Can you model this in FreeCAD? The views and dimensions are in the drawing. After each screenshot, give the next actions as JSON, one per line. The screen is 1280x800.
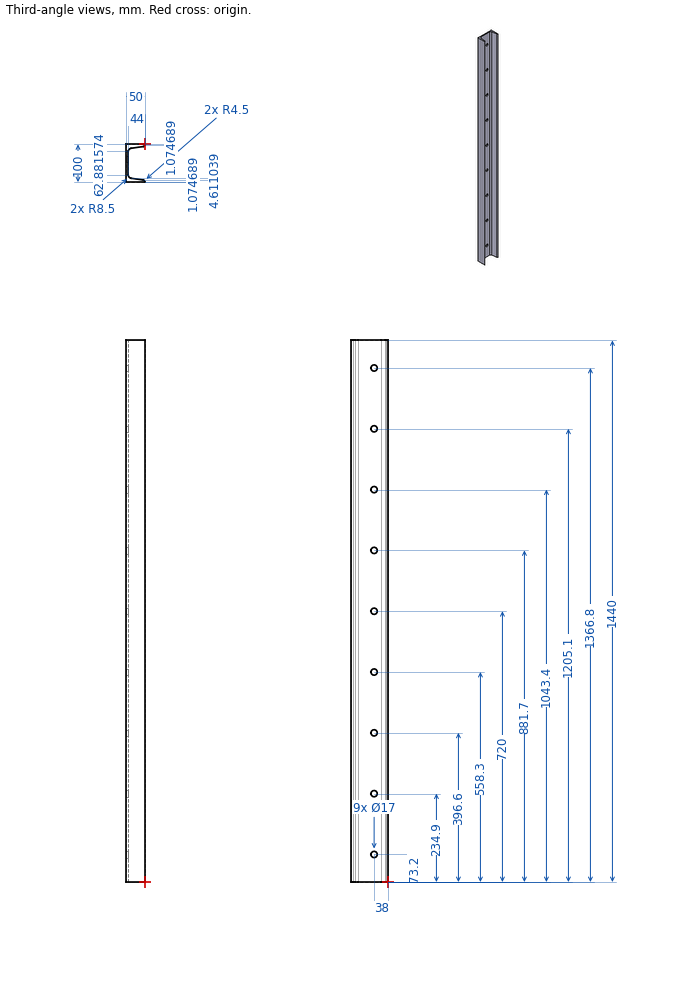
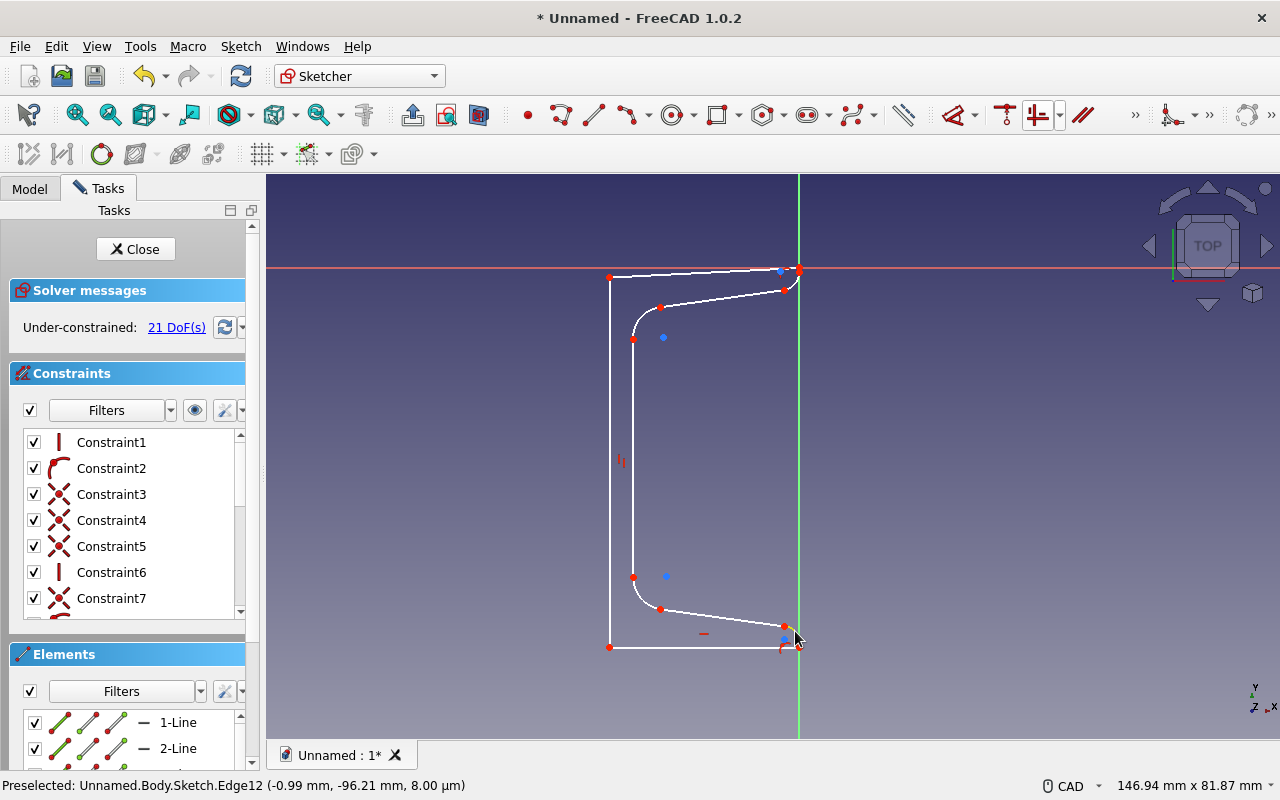
{"action": "left_click", "coordinate": [747, 621]}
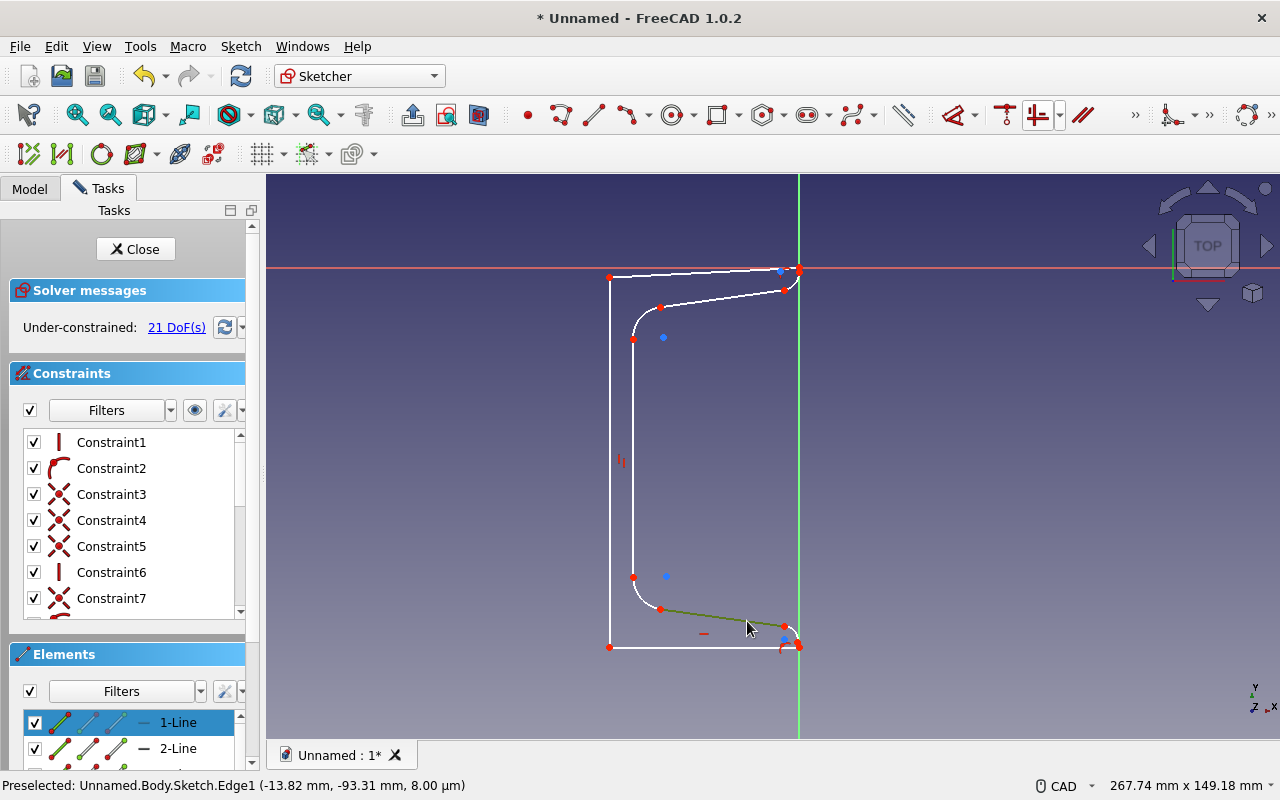
{"action": "left_click", "coordinate": [636, 591]}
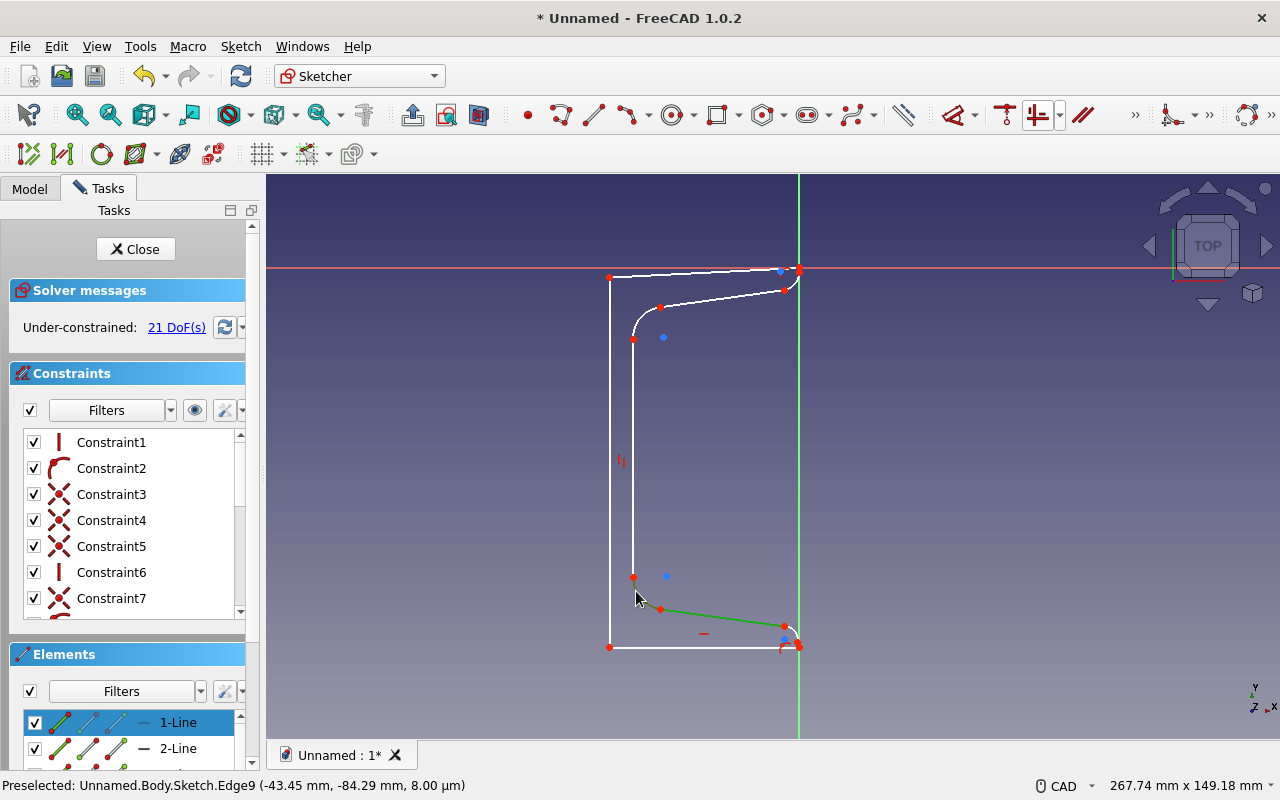
{"action": "key", "text": "t"}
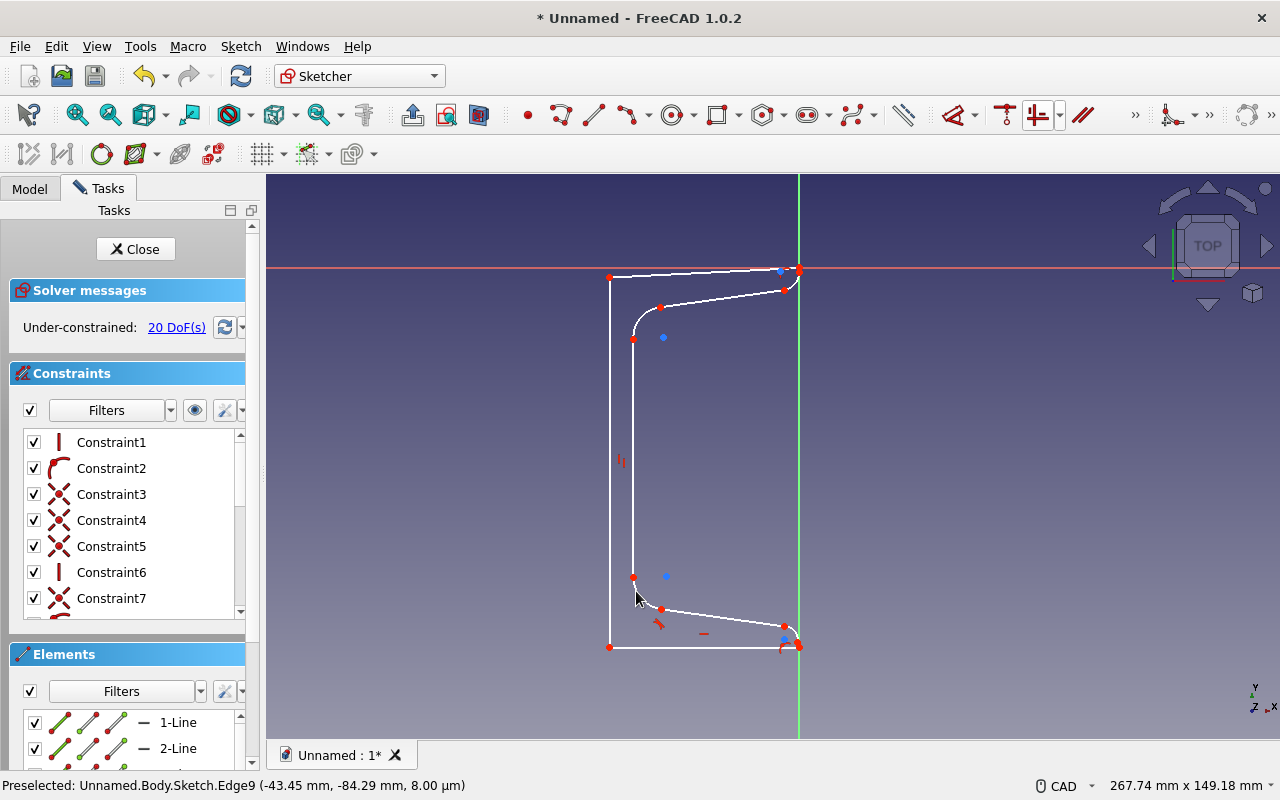
{"action": "left_click", "coordinate": [748, 621]}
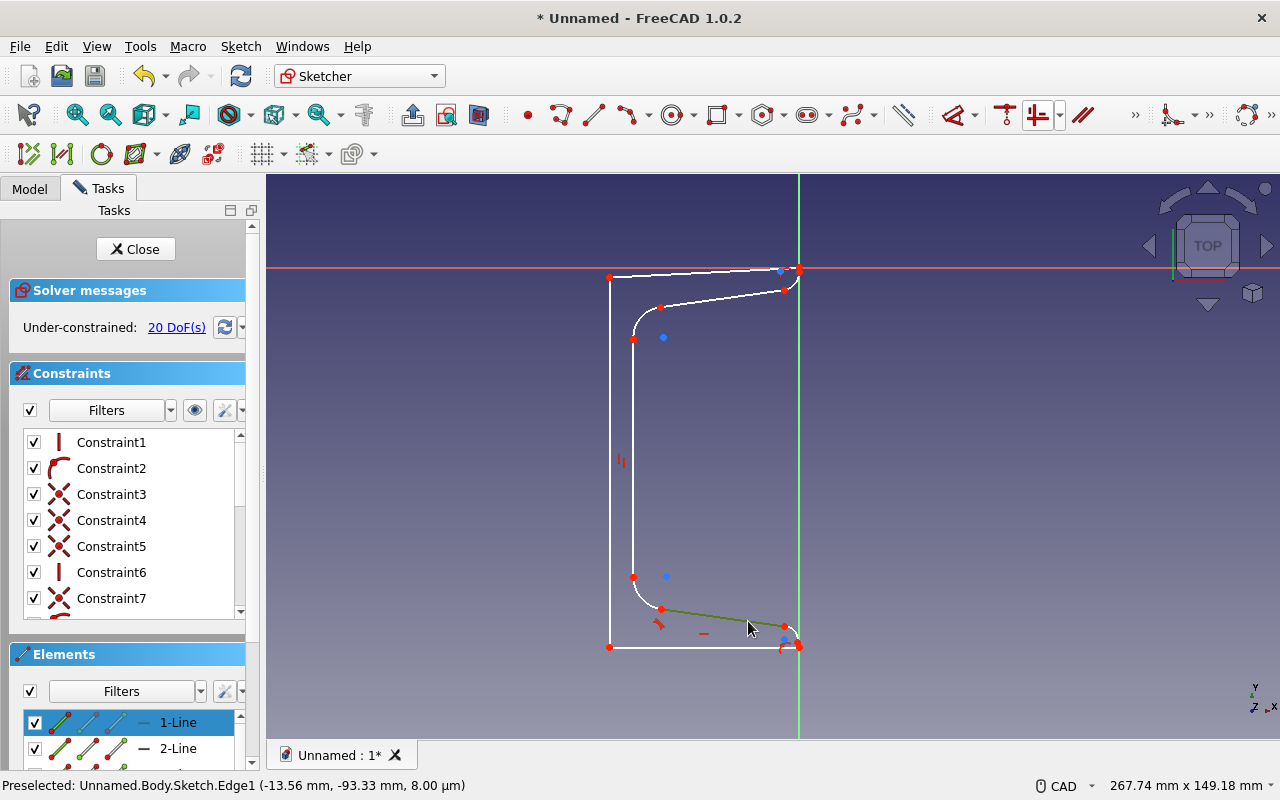
{"action": "scroll", "coordinate": [792, 628], "scroll_direction": "up", "scroll_amount": 4}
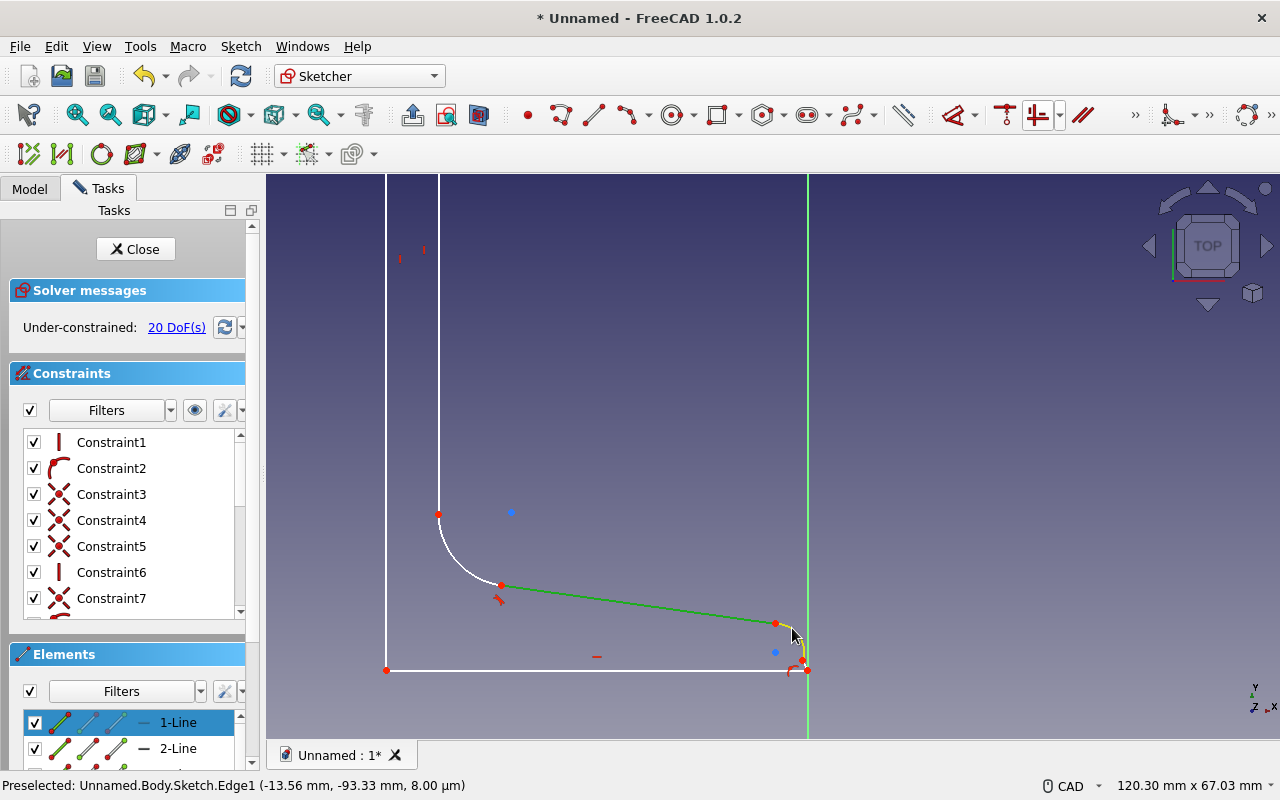
{"action": "left_click", "coordinate": [790, 628]}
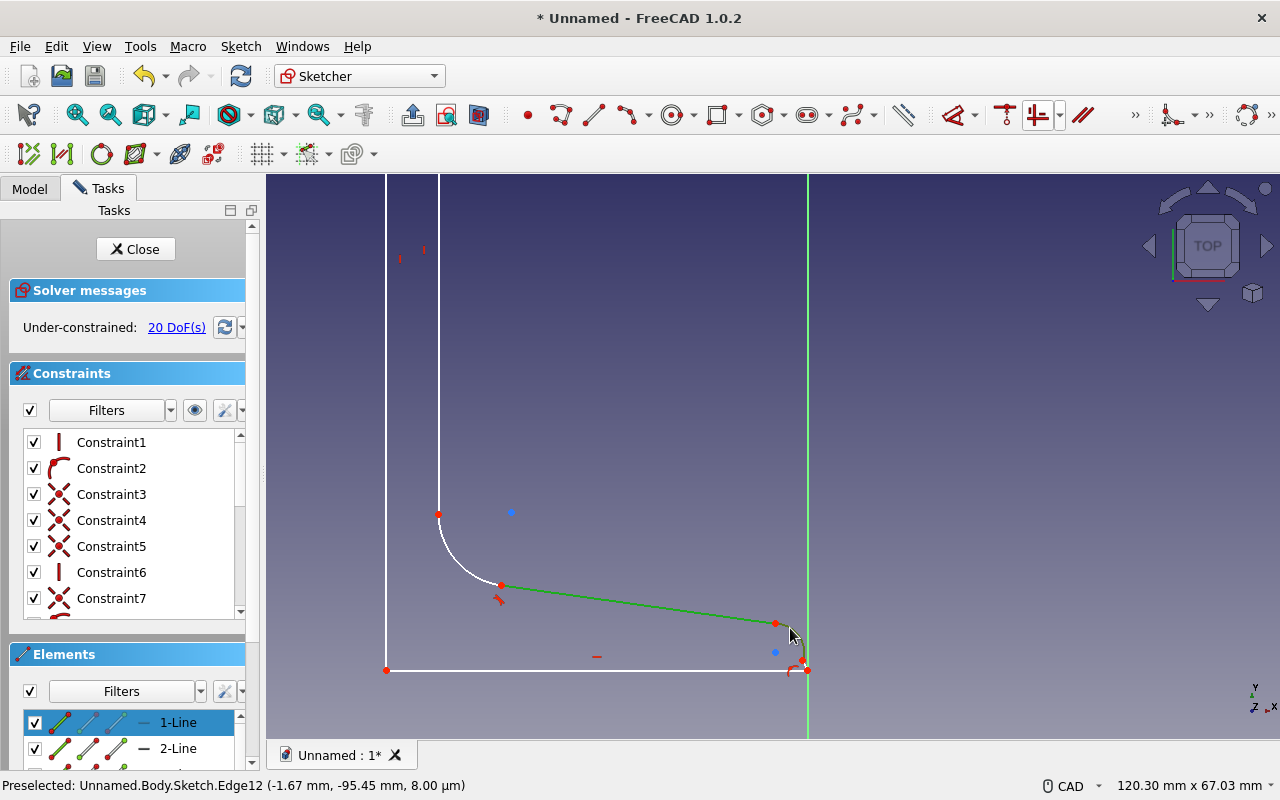
{"action": "key", "text": "t"}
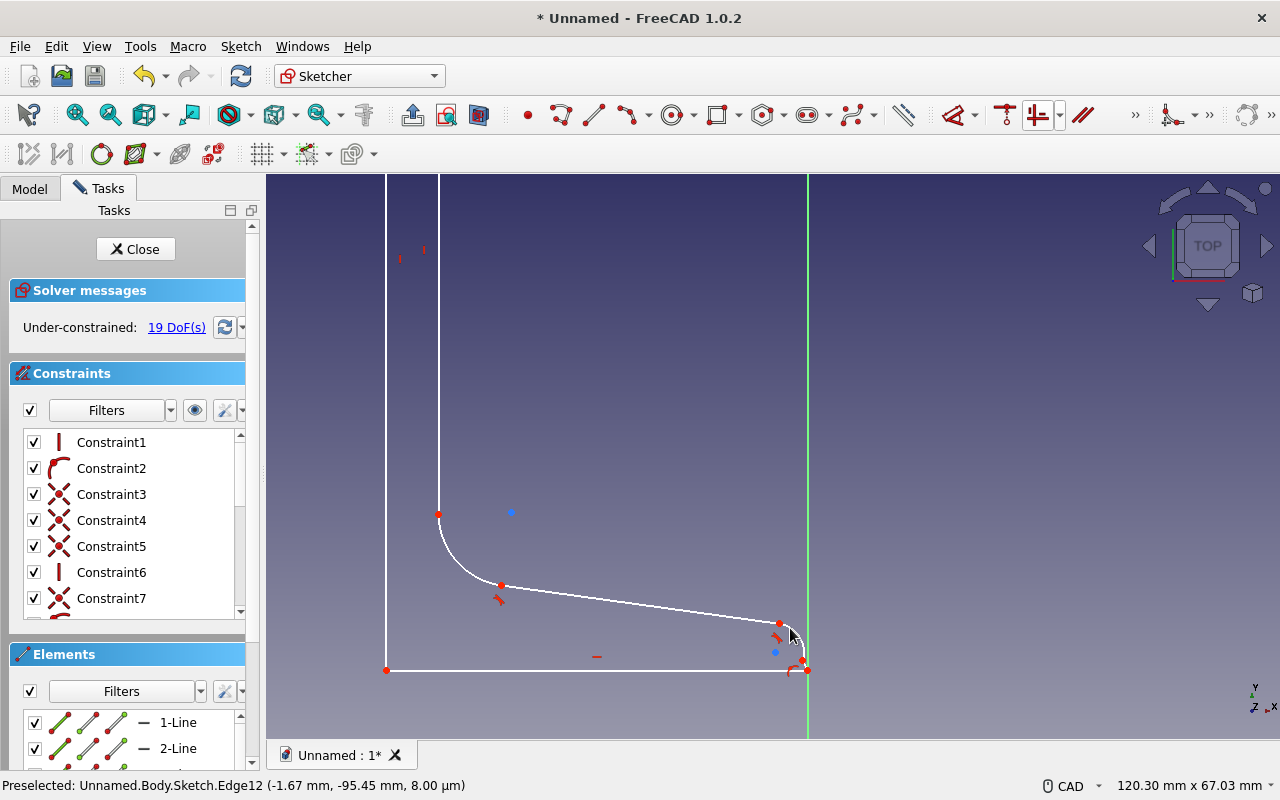
{"action": "left_click", "coordinate": [439, 355]}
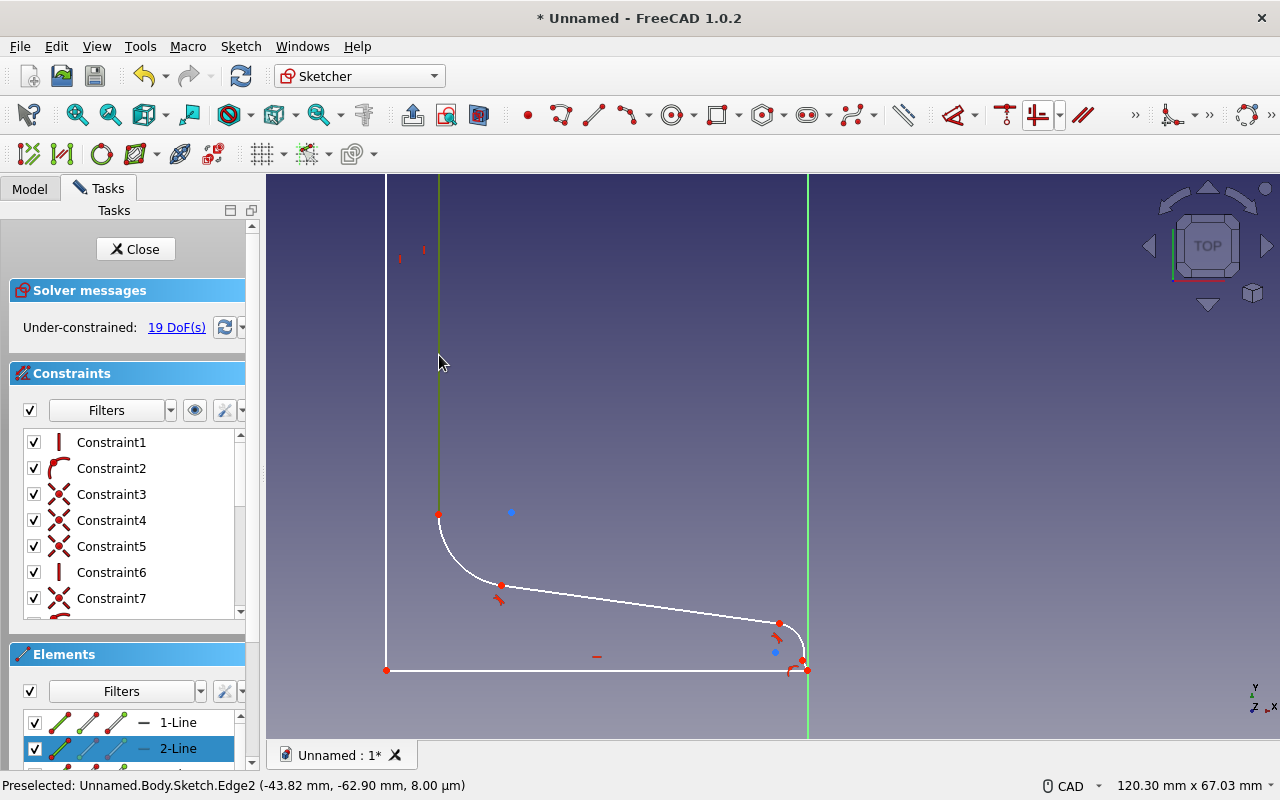
{"action": "left_click", "coordinate": [446, 544]}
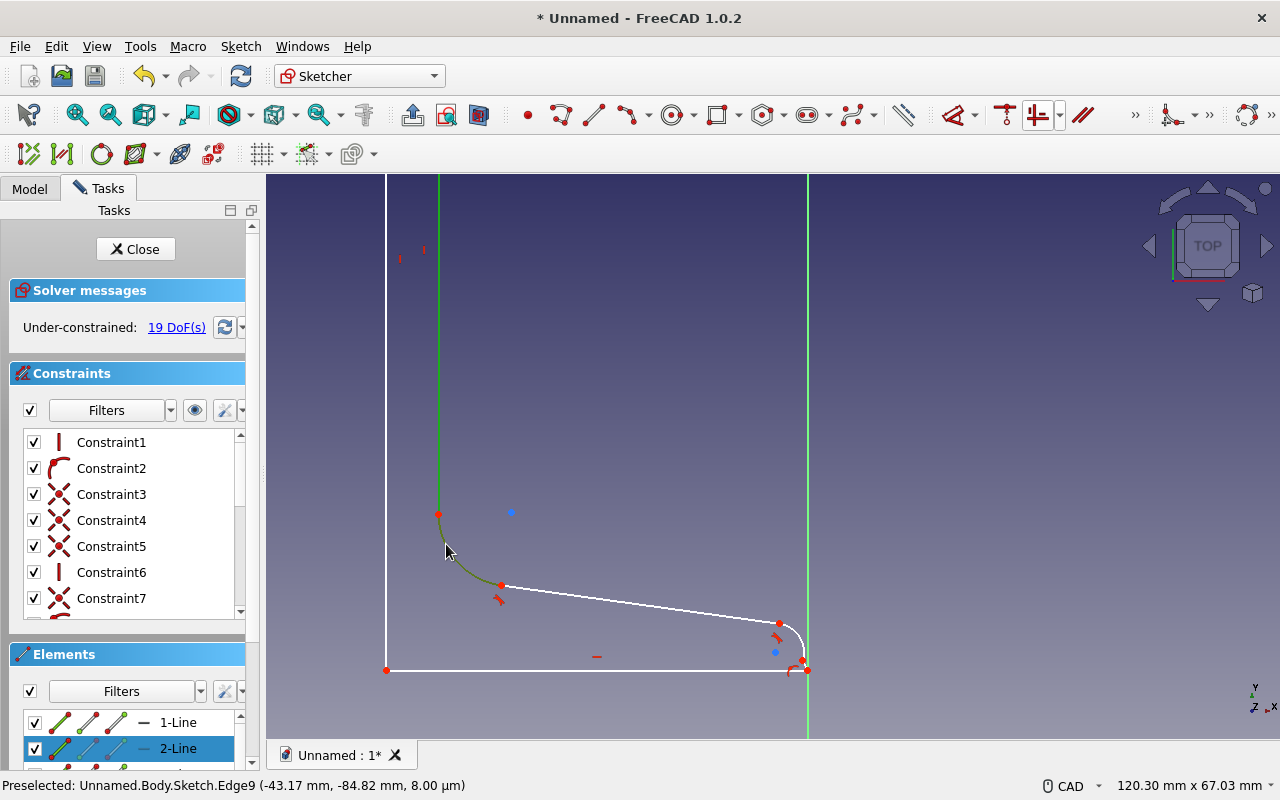
{"action": "key", "text": "t"}